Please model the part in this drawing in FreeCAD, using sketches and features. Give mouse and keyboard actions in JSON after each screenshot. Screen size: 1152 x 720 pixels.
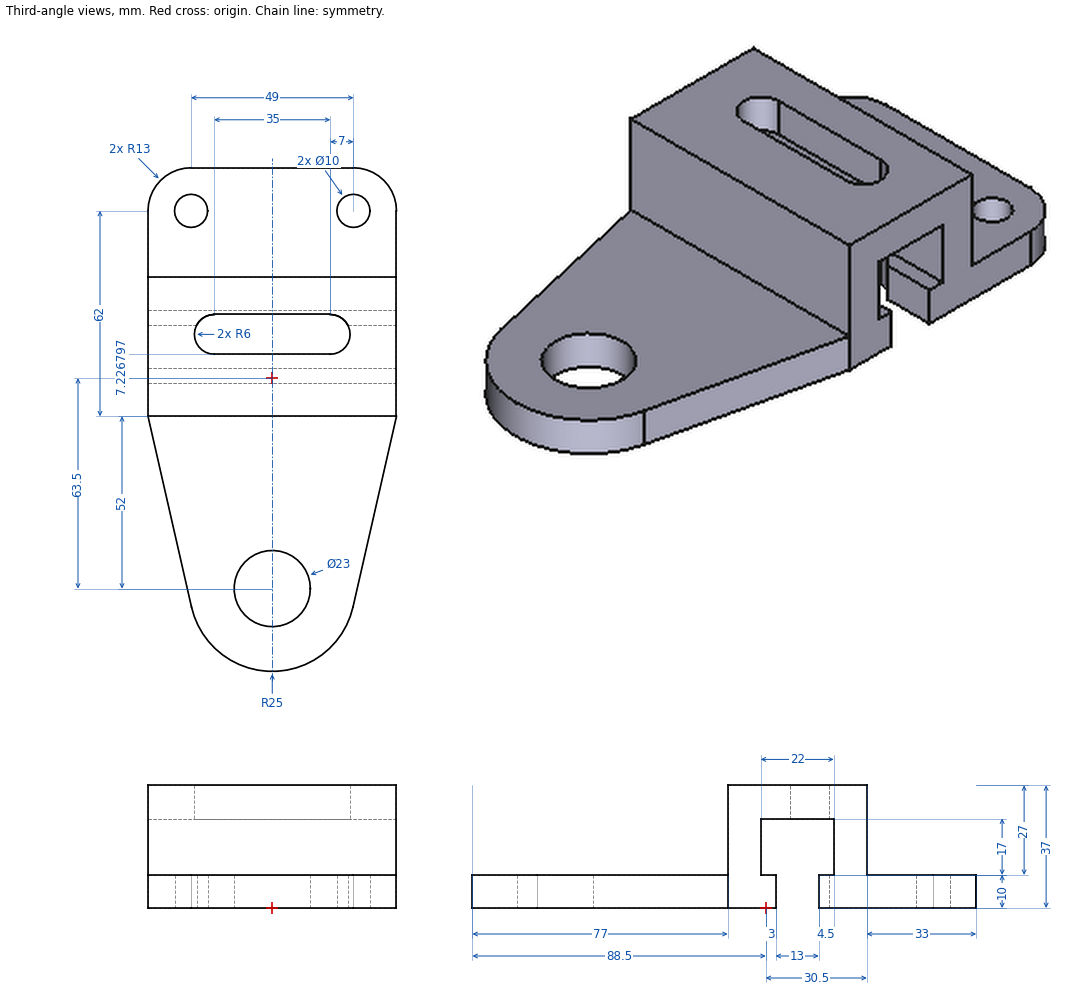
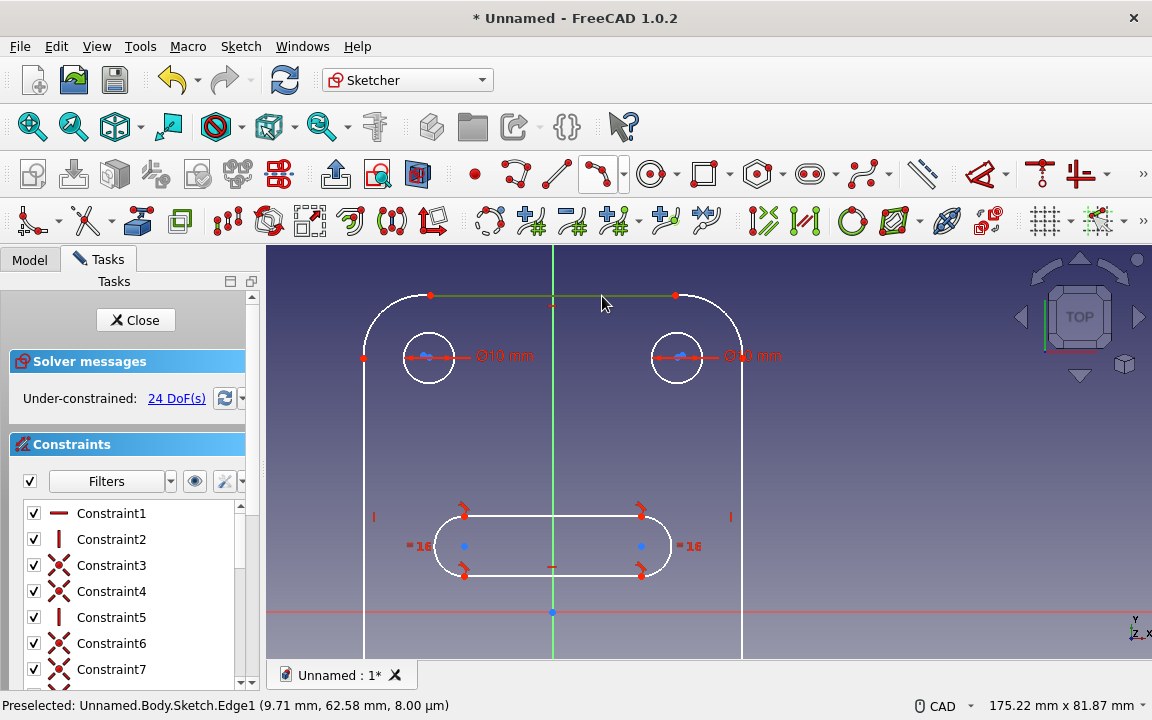
{"action": "left_click", "coordinate": [400, 300]}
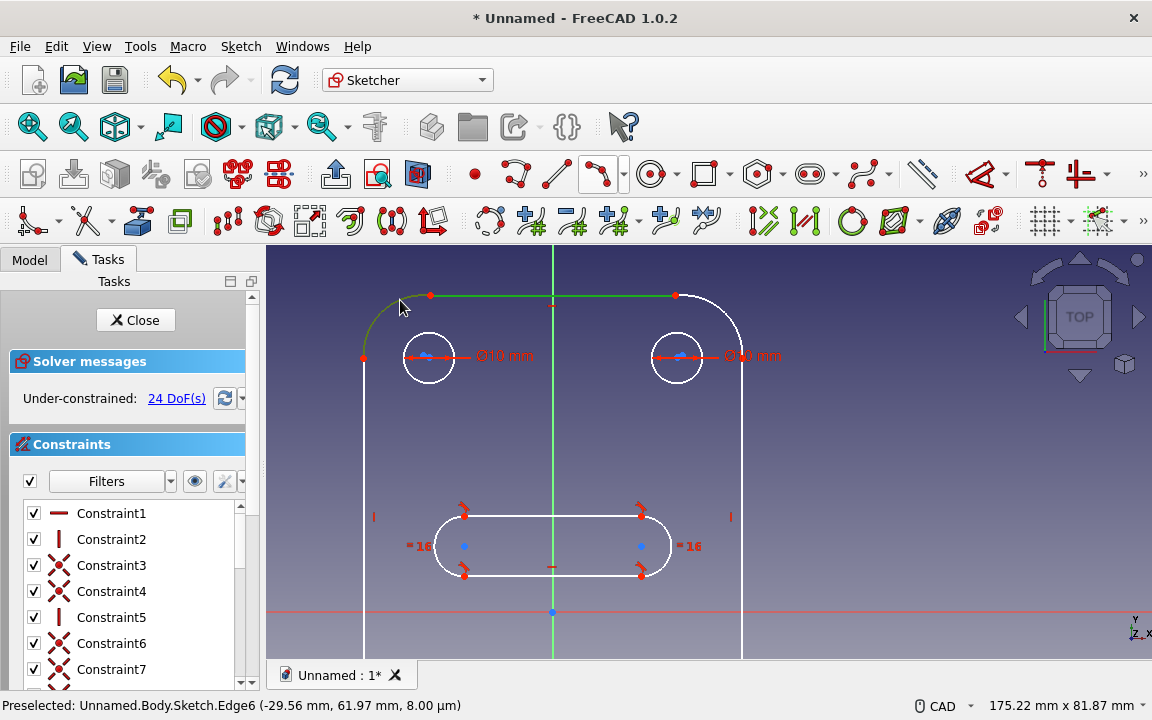
{"action": "key", "text": "t"}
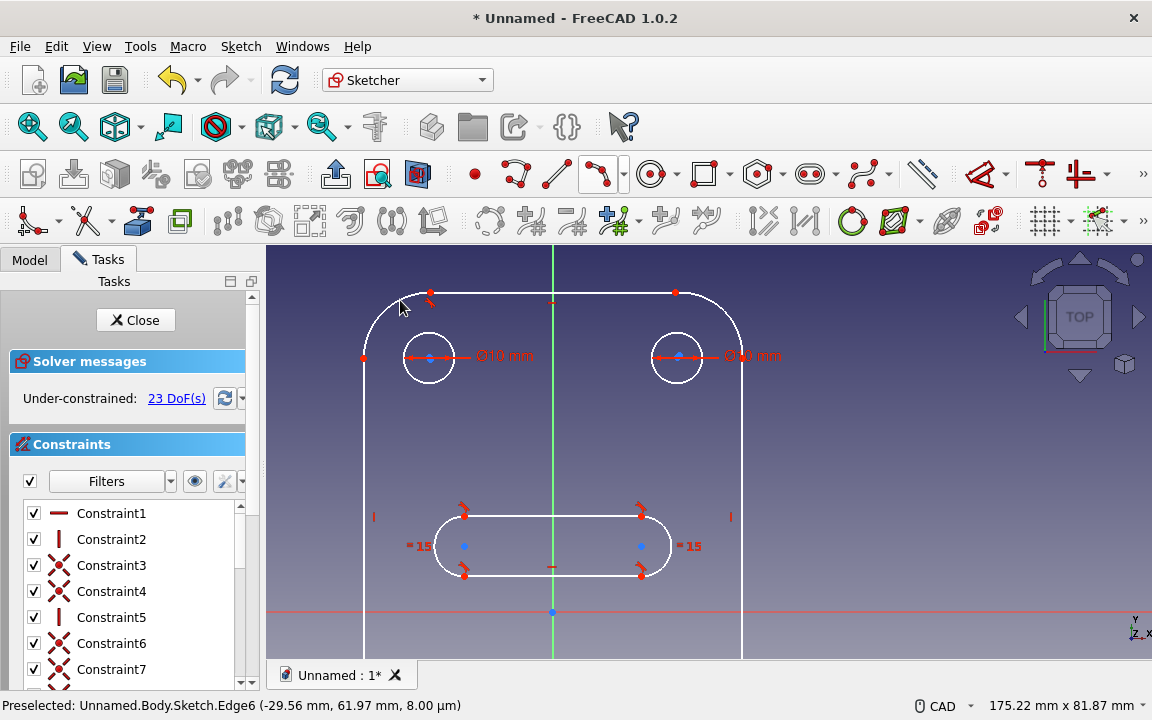
{"action": "left_click", "coordinate": [602, 293]}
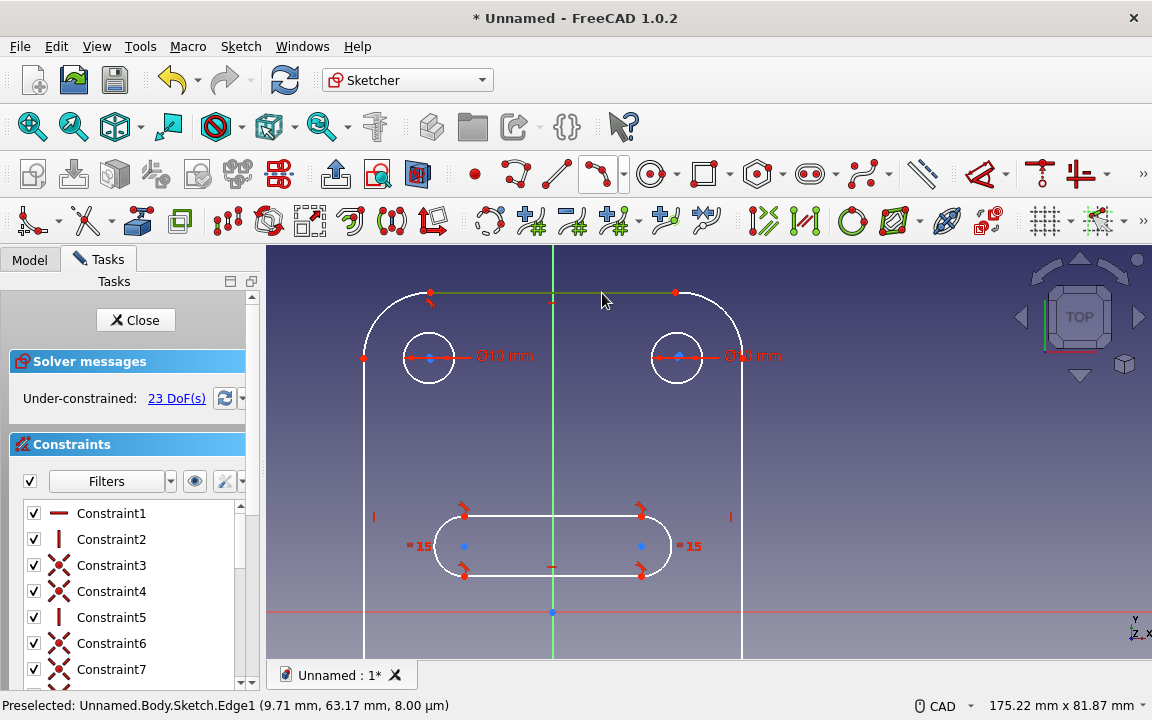
{"action": "left_click", "coordinate": [736, 328]}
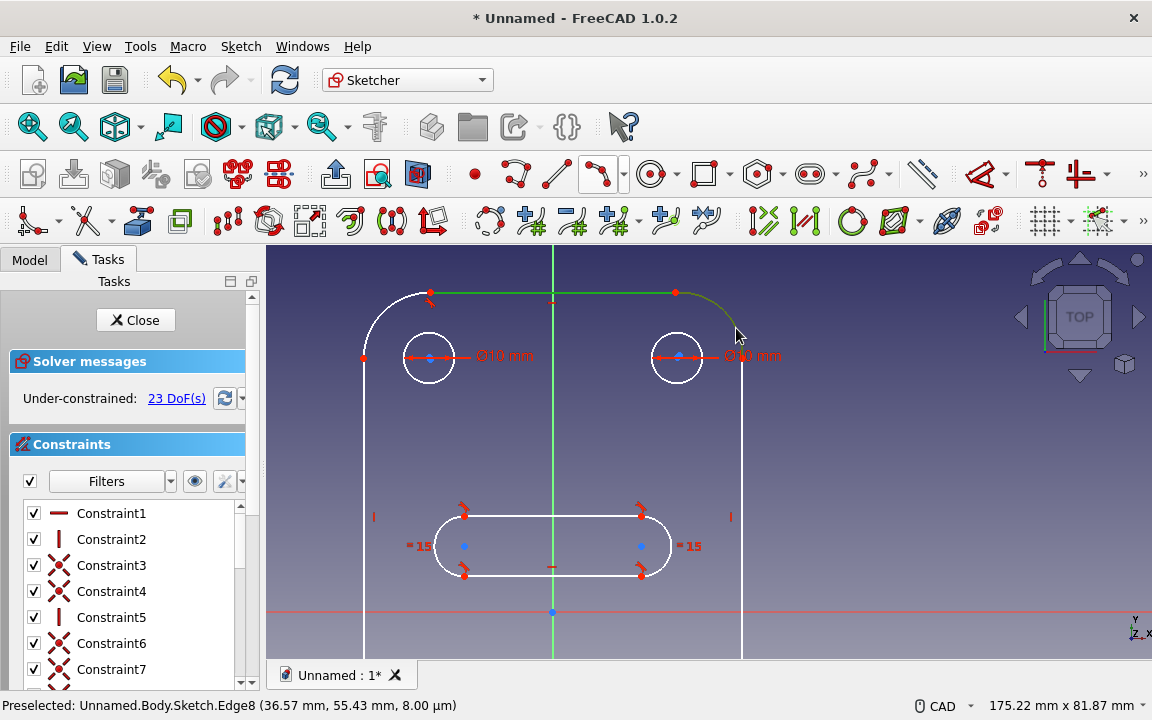
{"action": "key", "text": "t"}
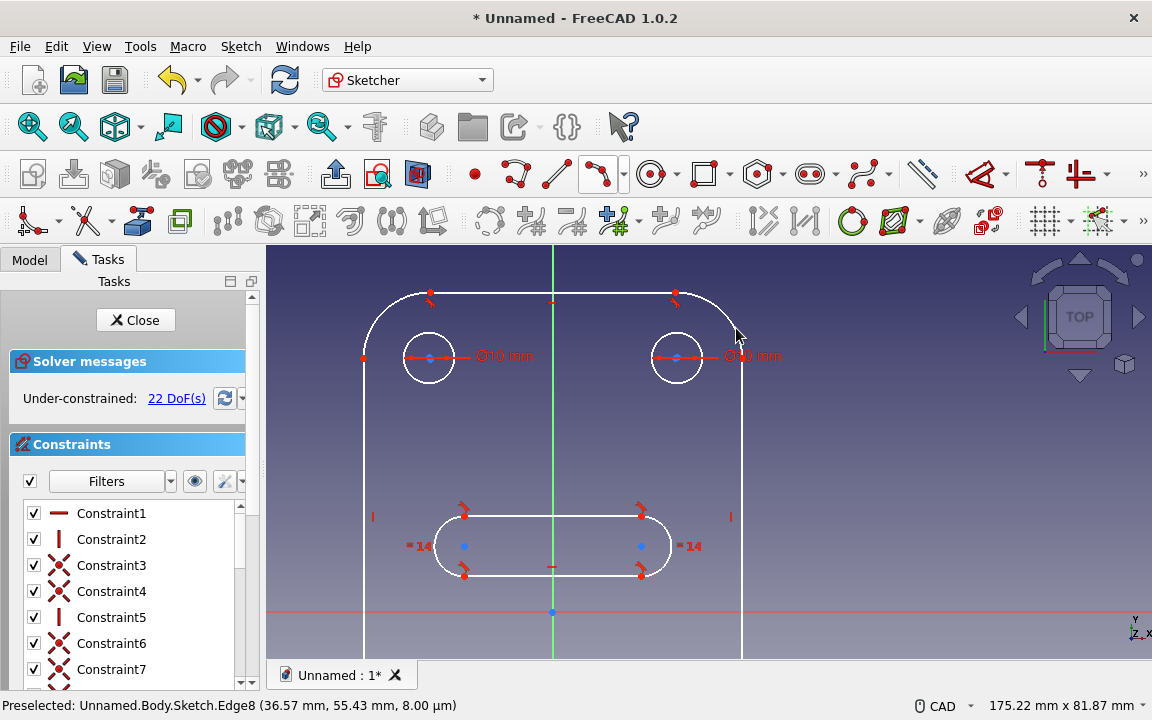
{"action": "left_click", "coordinate": [364, 453]}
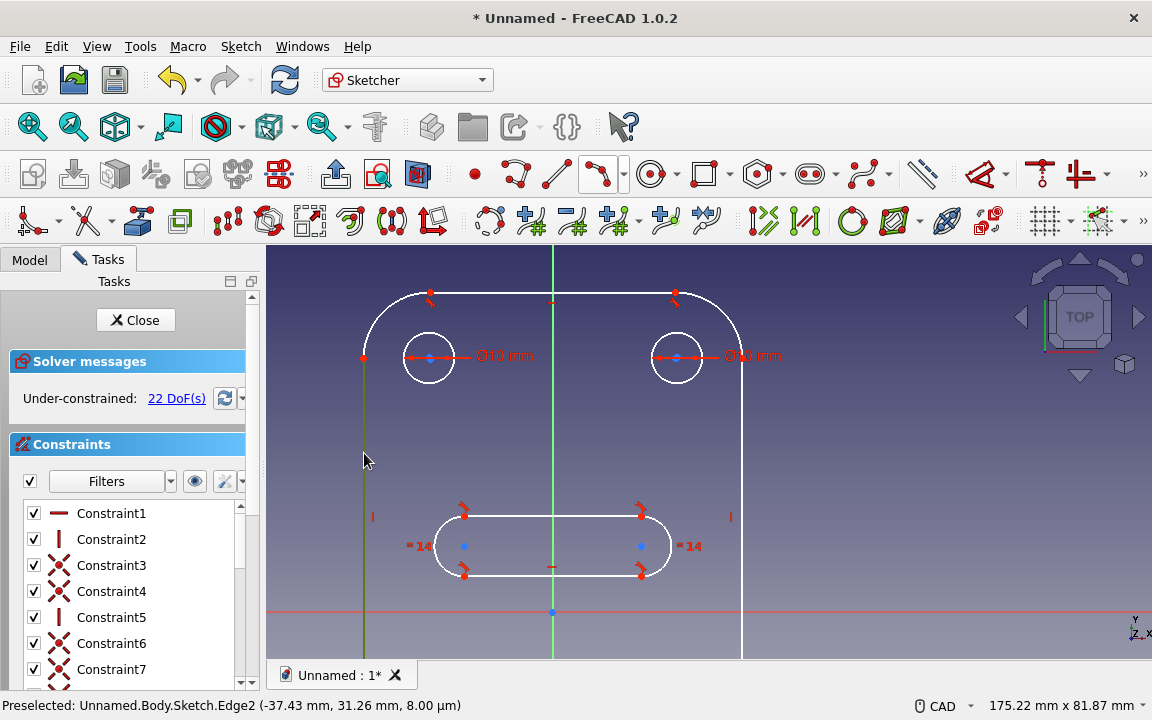
{"action": "left_click", "coordinate": [400, 300]}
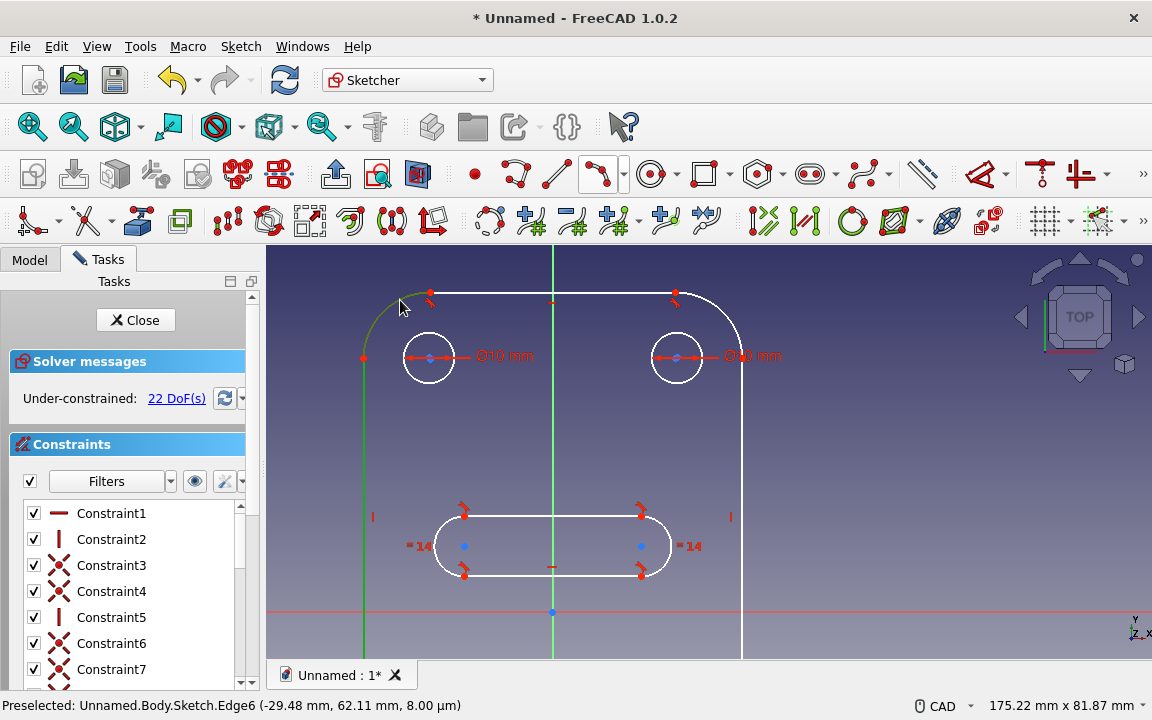
{"action": "key", "text": "t"}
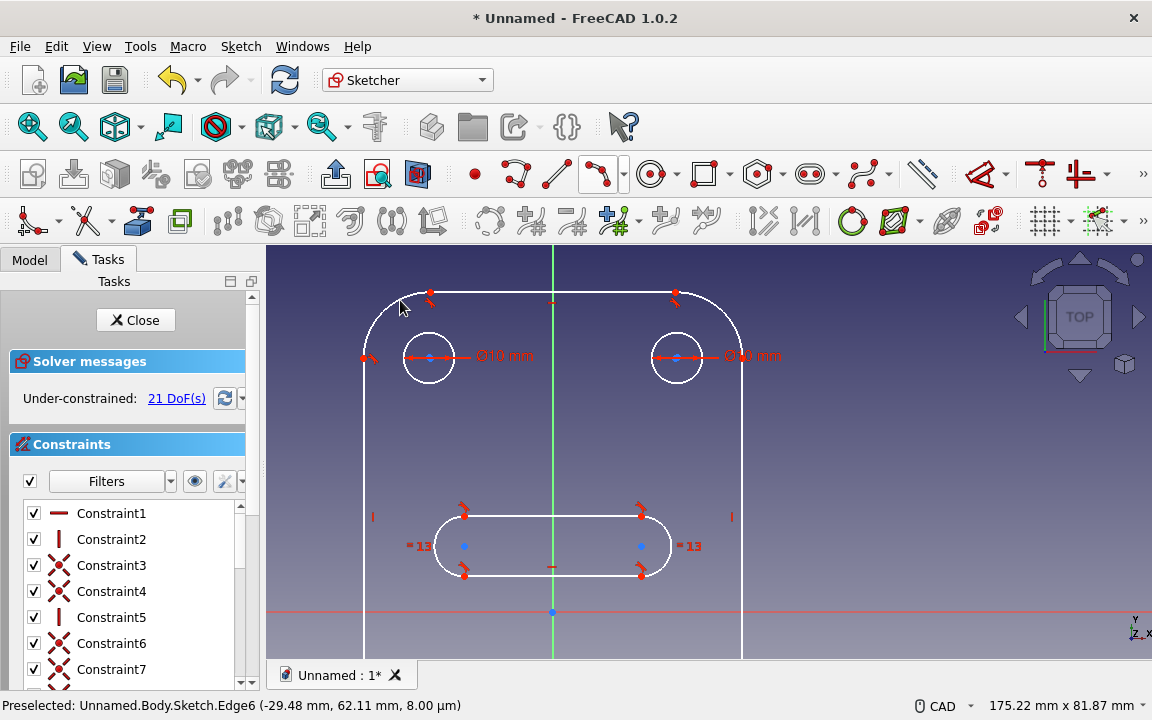
{"action": "scroll", "coordinate": [678, 356], "scroll_direction": "down", "scroll_amount": 6}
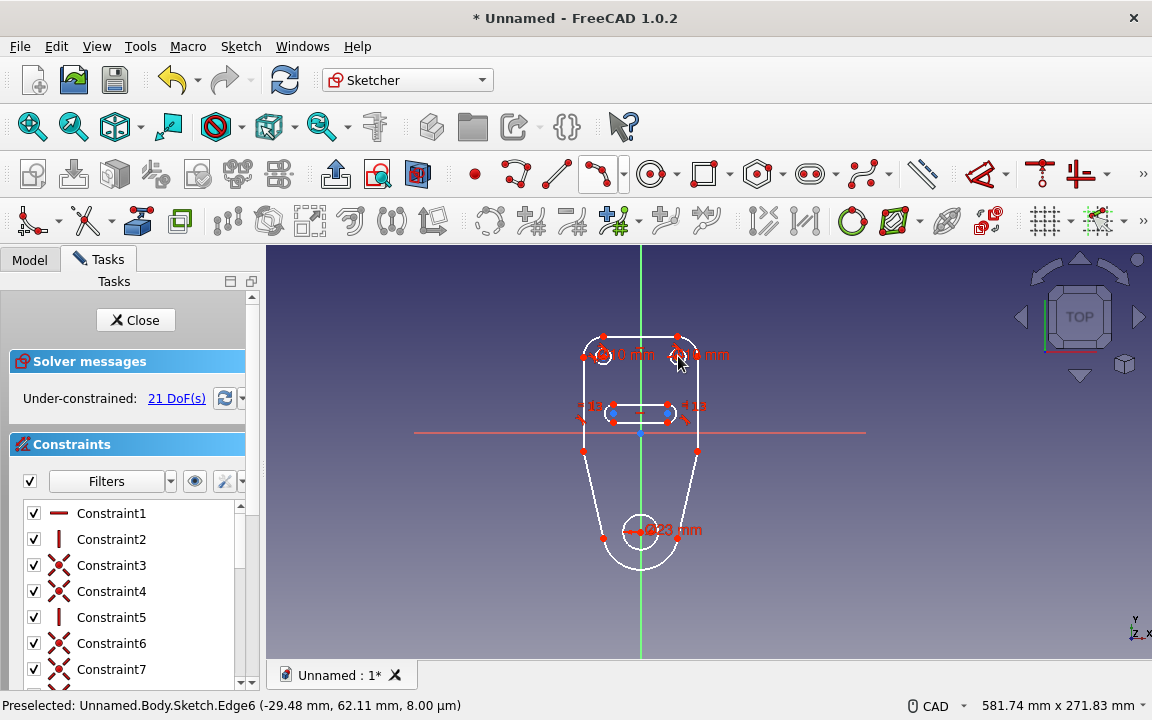
{"action": "left_click", "coordinate": [590, 478]}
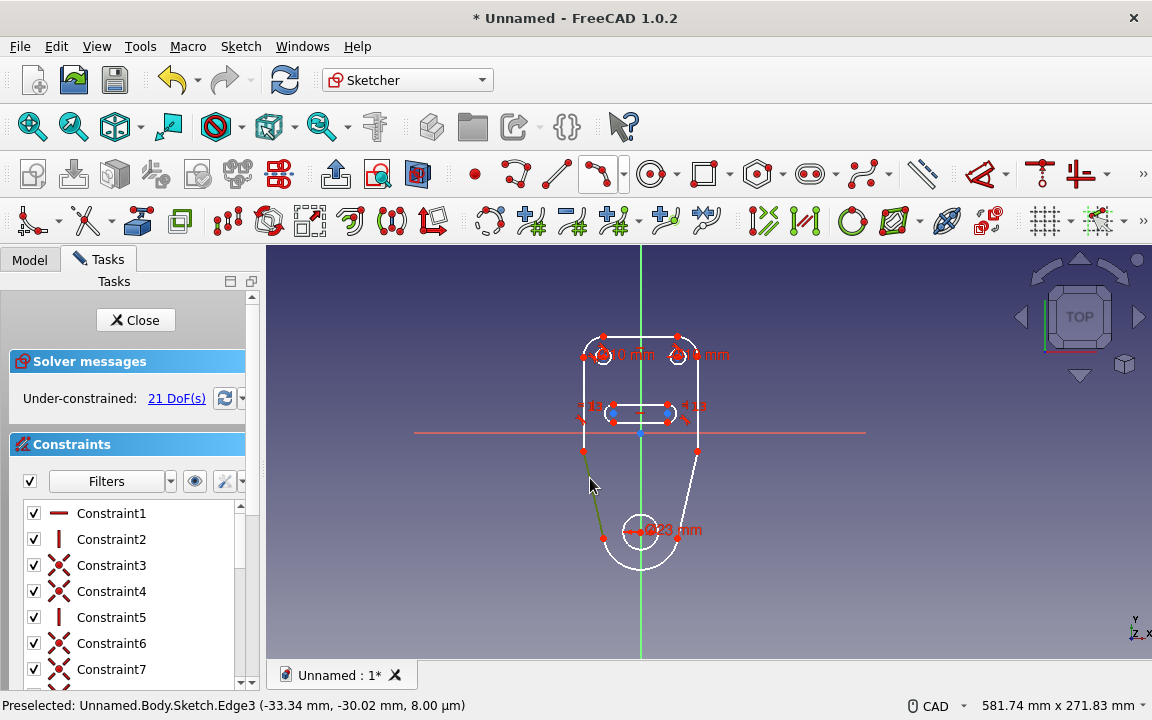
{"action": "left_click", "coordinate": [621, 564]}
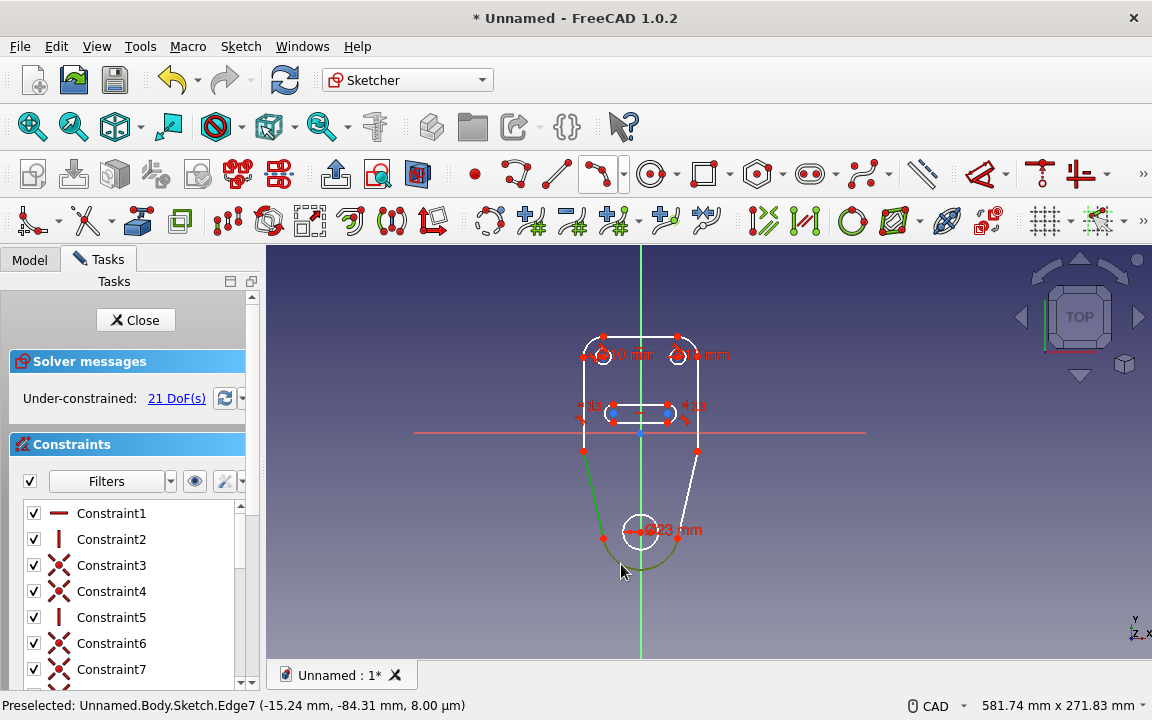
{"action": "key", "text": "t"}